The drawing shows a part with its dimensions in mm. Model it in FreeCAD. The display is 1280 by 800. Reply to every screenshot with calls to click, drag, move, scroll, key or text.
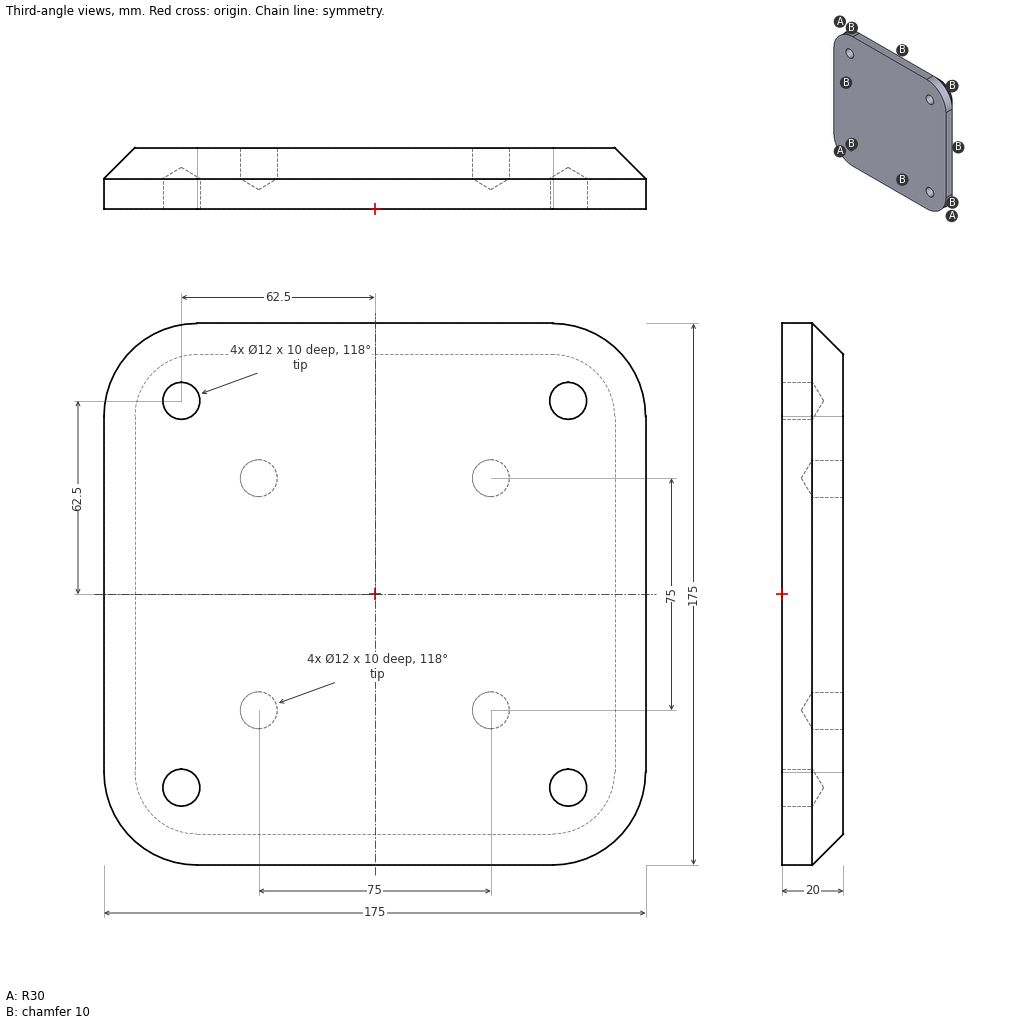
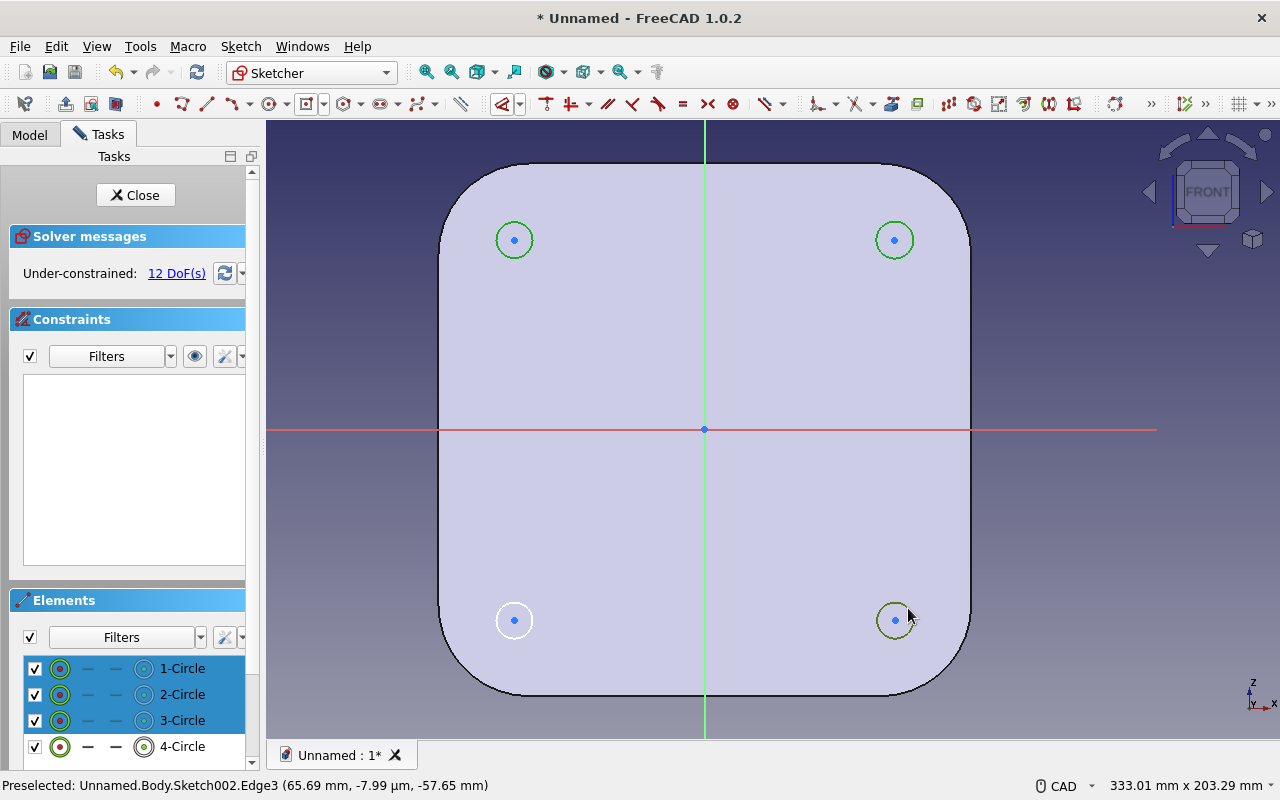
click(527, 608)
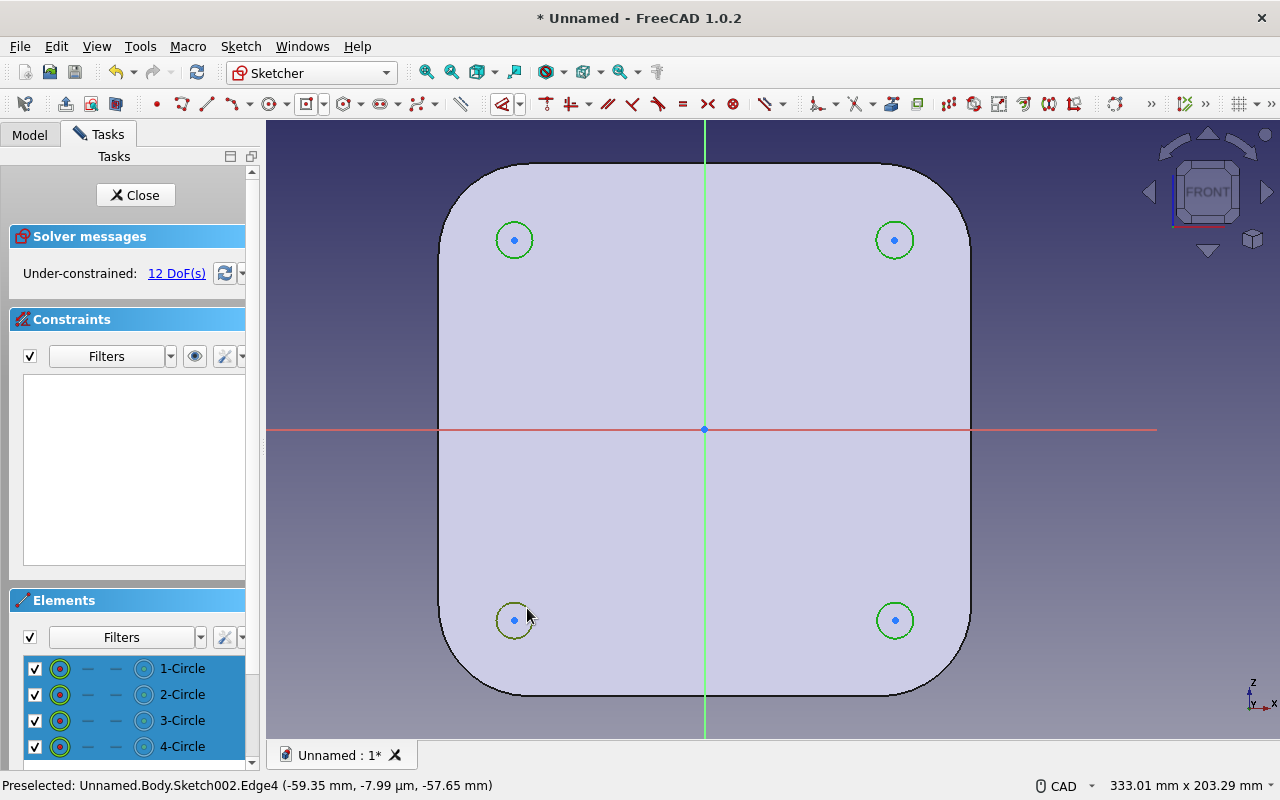
click(683, 104)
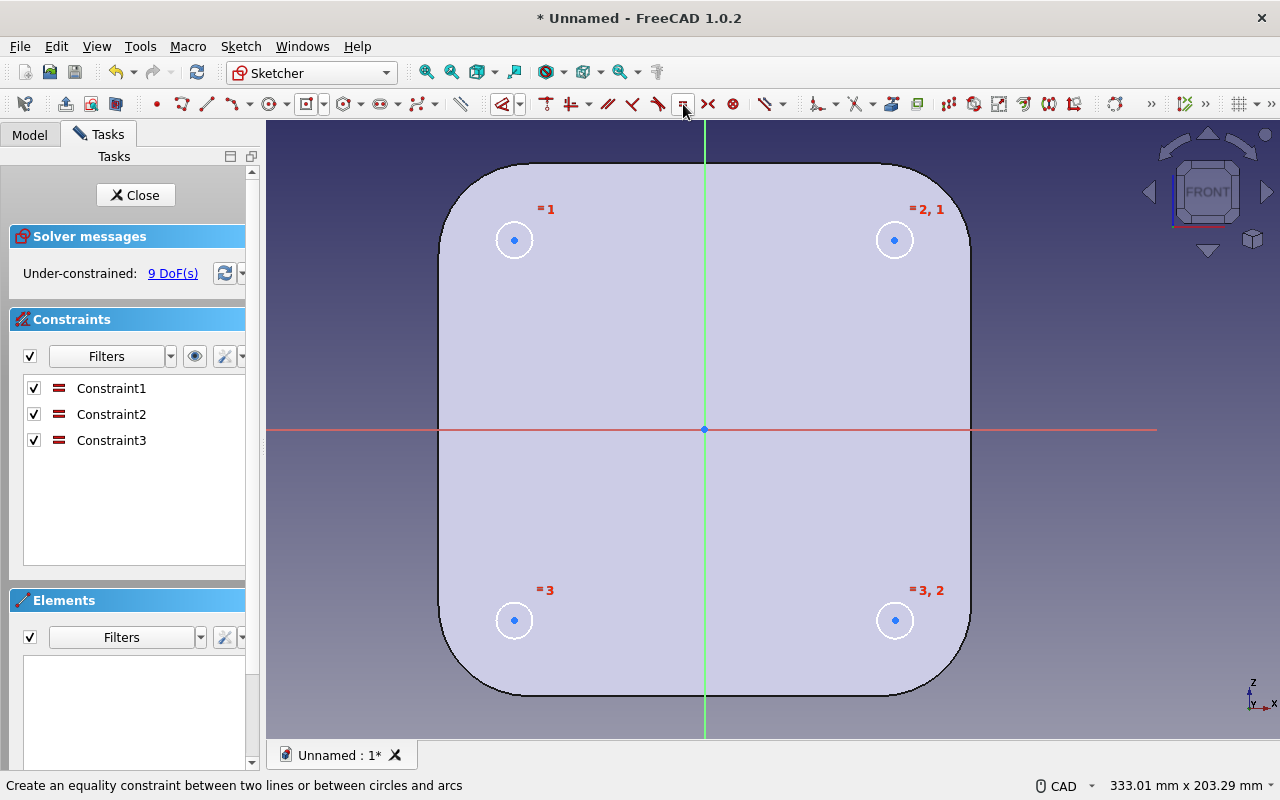
click(514, 240)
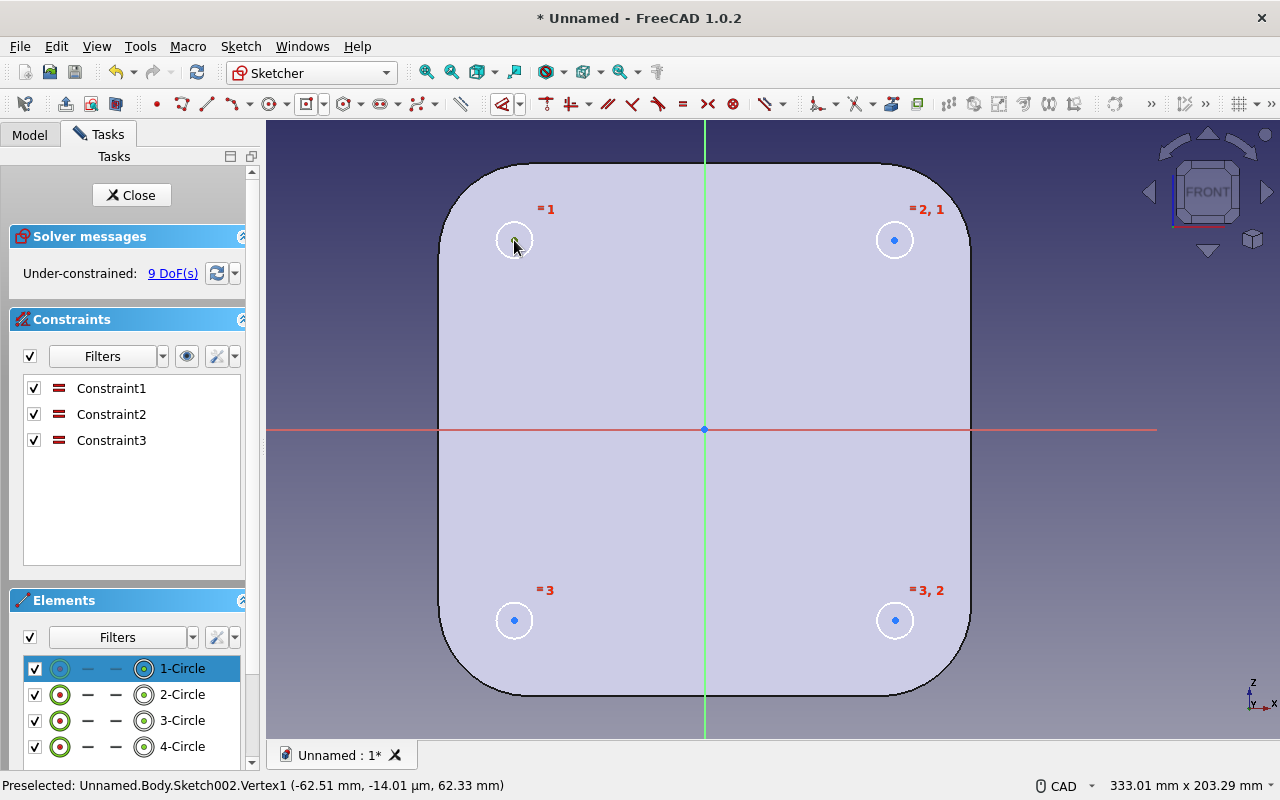
click(895, 240)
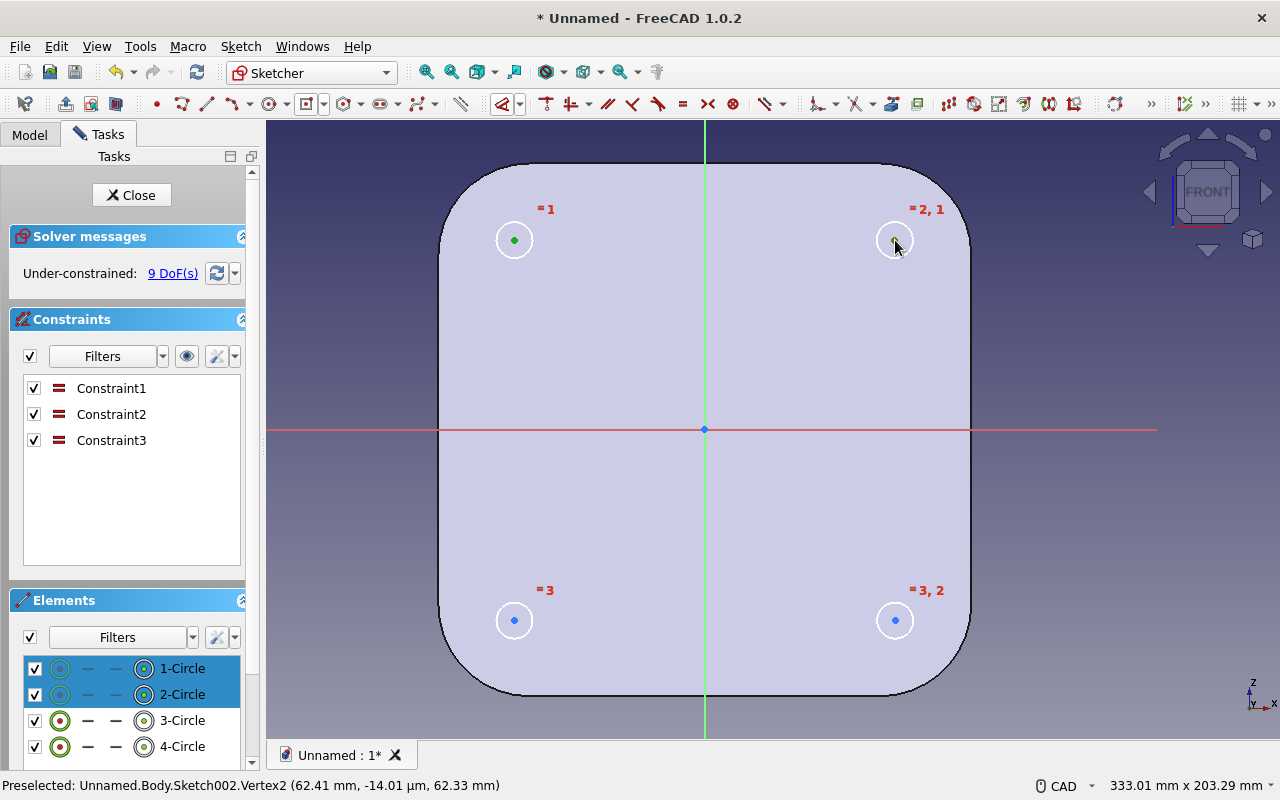
click(705, 671)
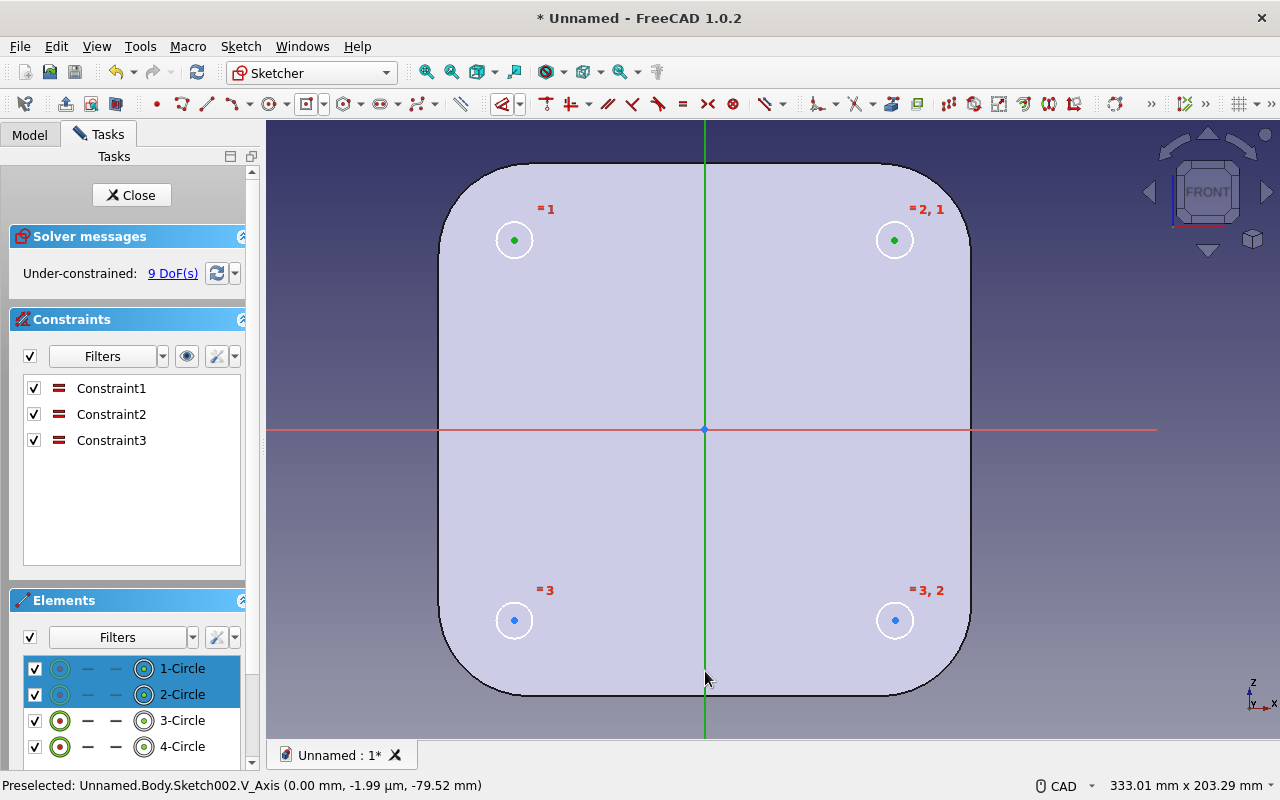
click(708, 104)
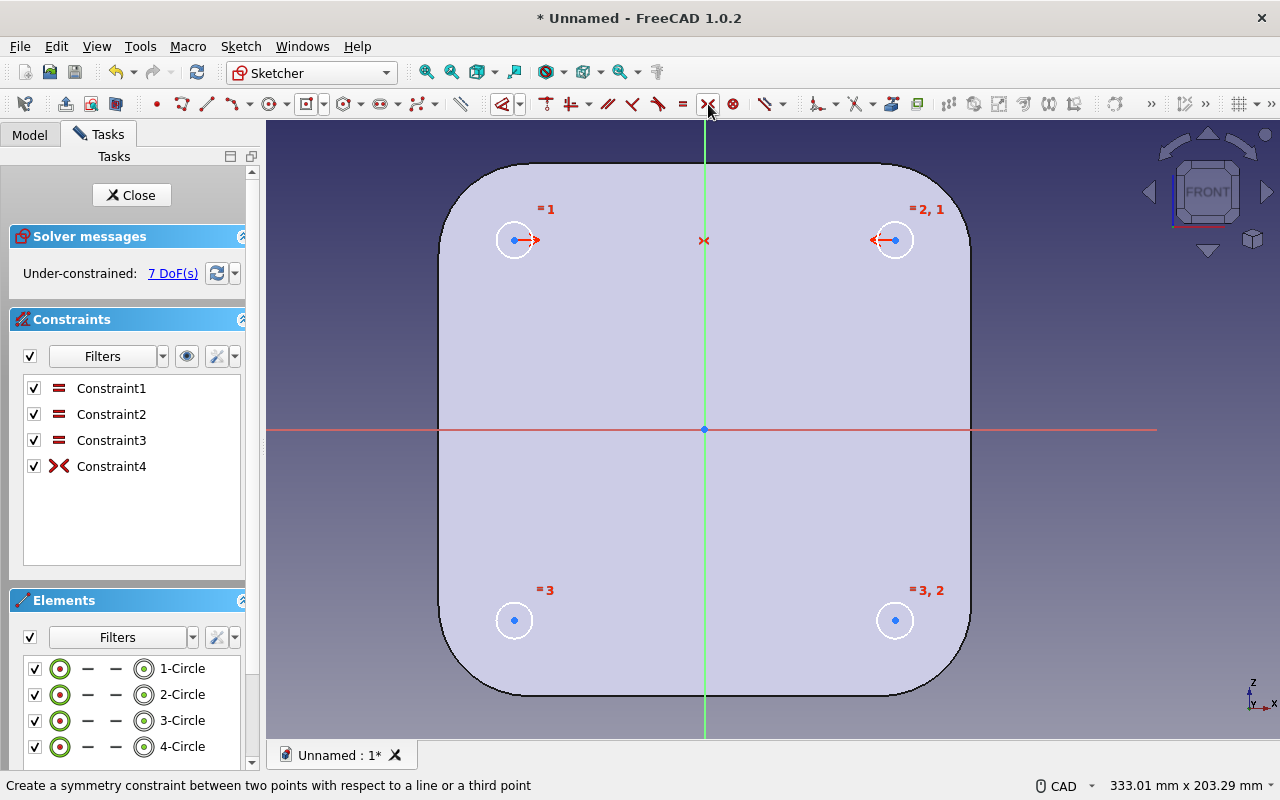
click(895, 240)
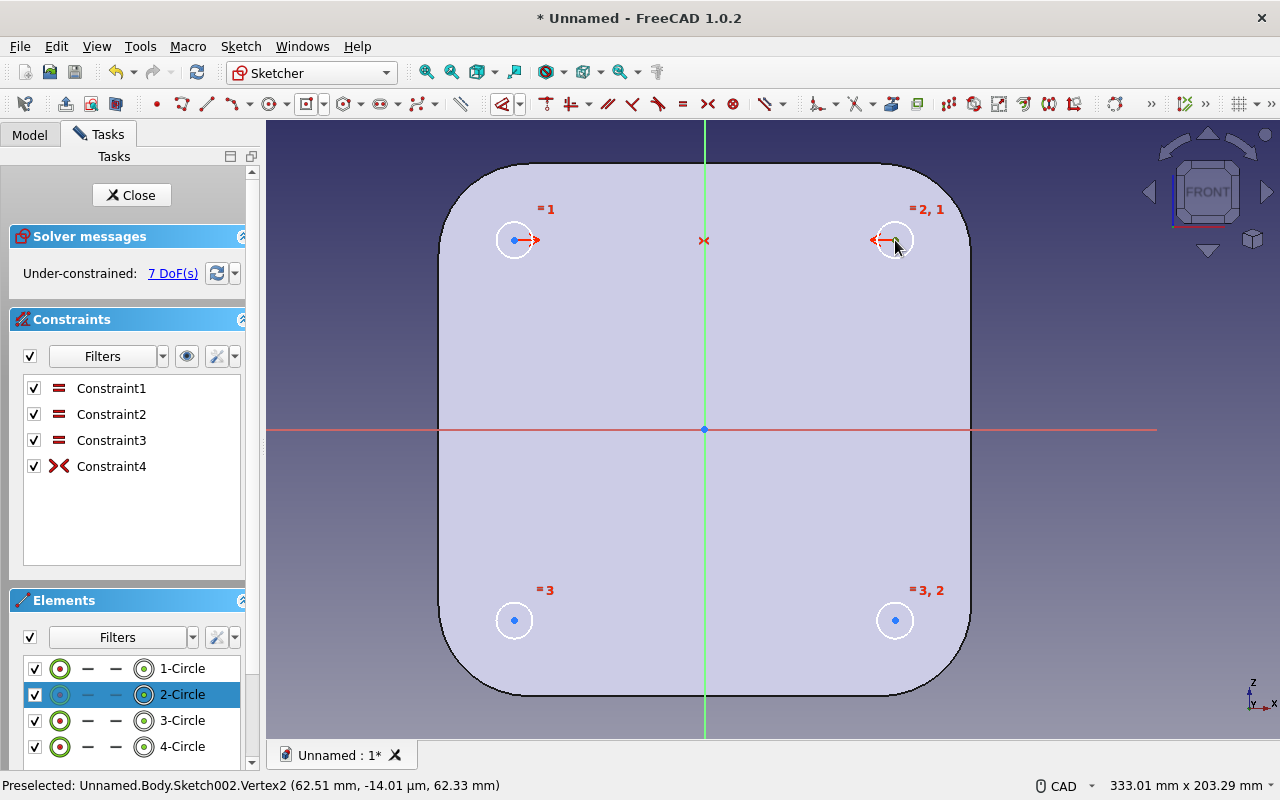
click(895, 621)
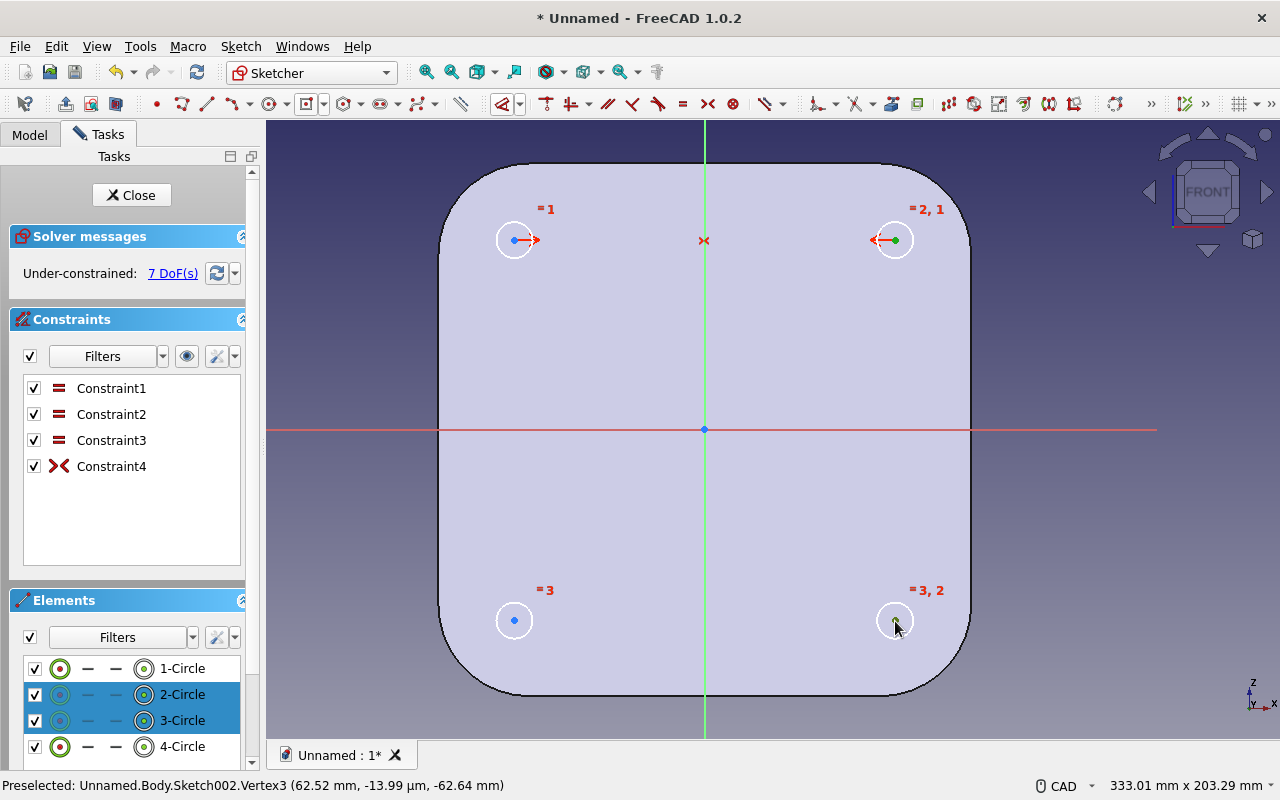
click(353, 430)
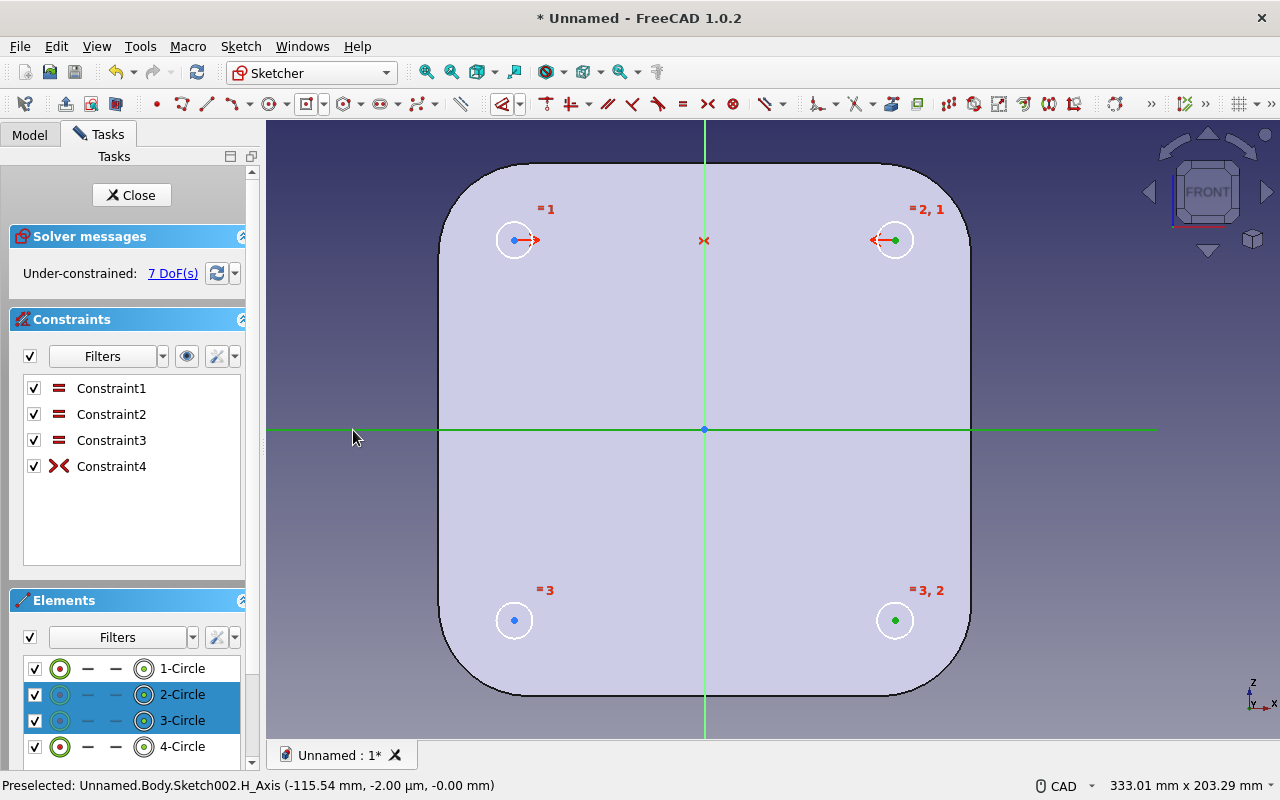
click(708, 104)